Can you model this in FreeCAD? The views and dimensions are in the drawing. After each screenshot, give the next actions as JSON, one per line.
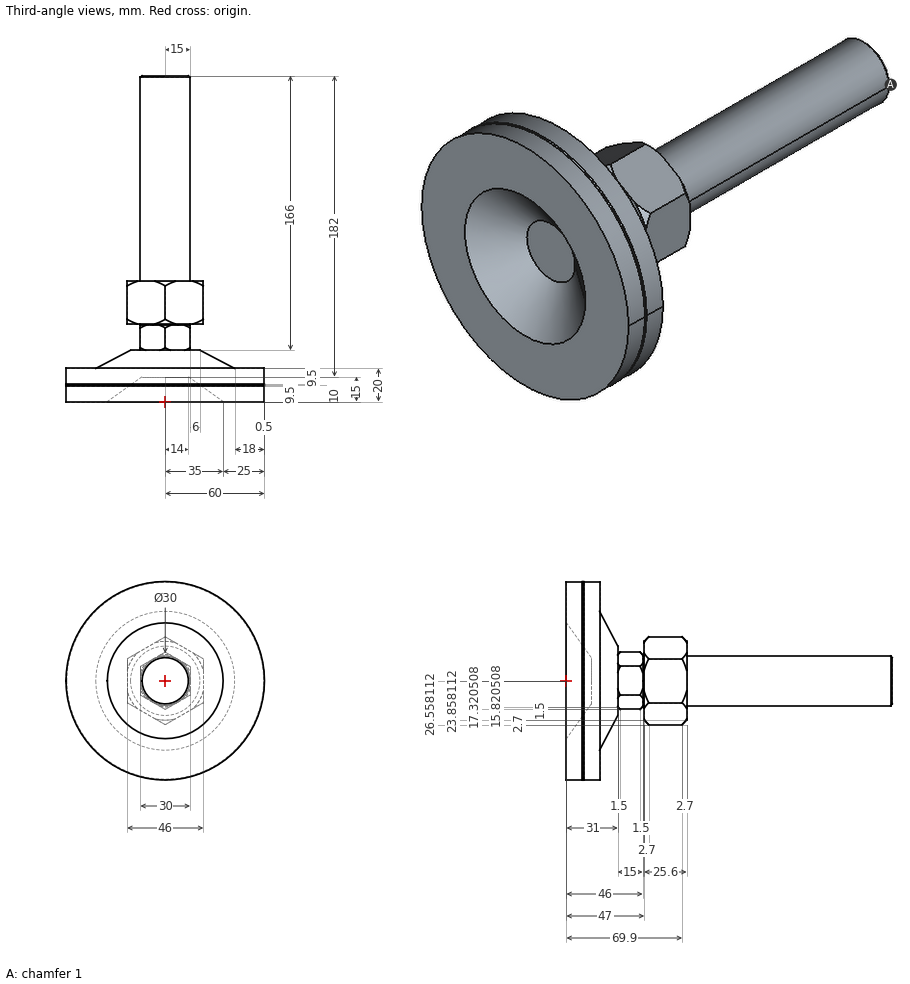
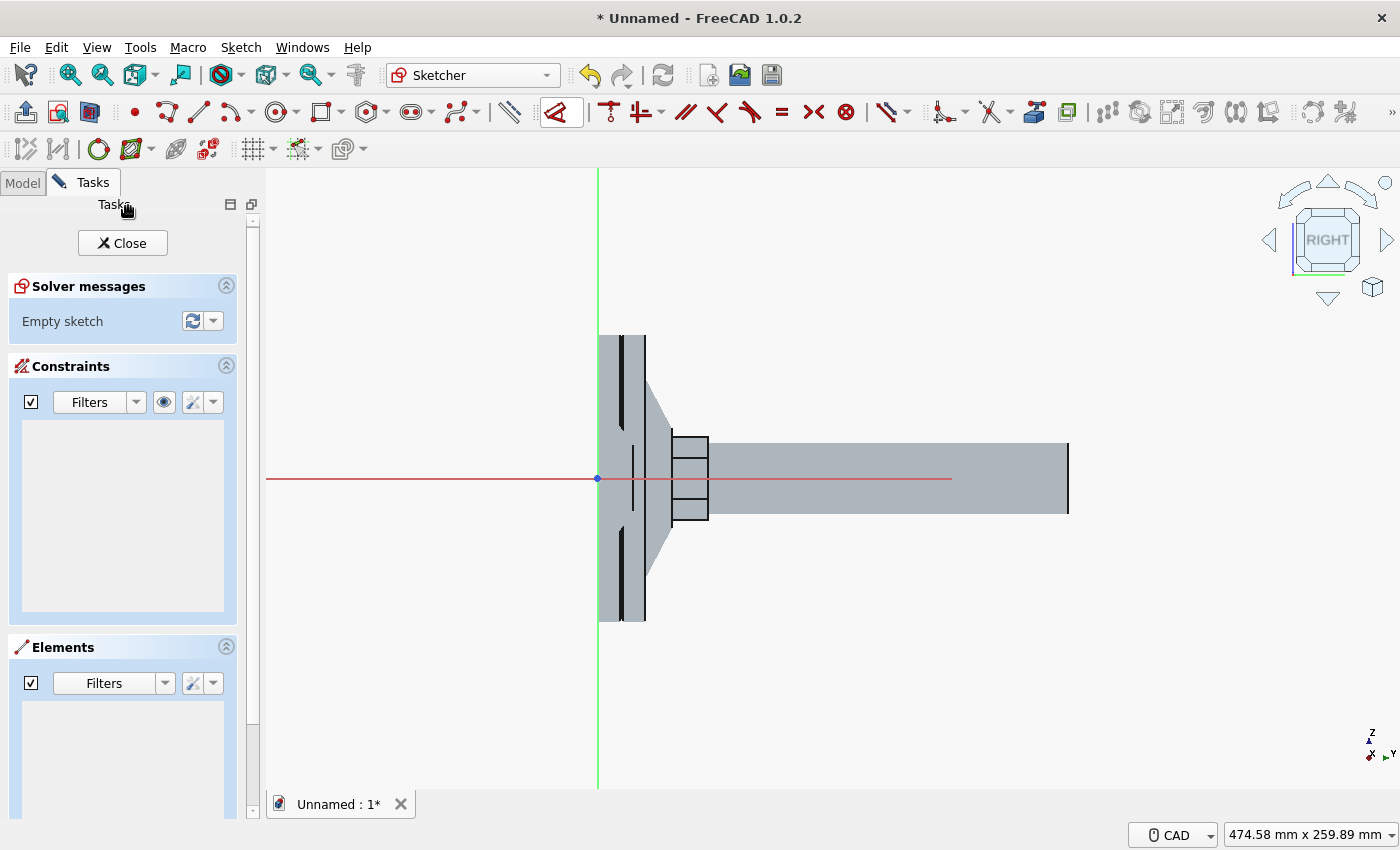
{"action": "scroll", "coordinate": [686, 520], "scroll_direction": "up", "scroll_amount": 15}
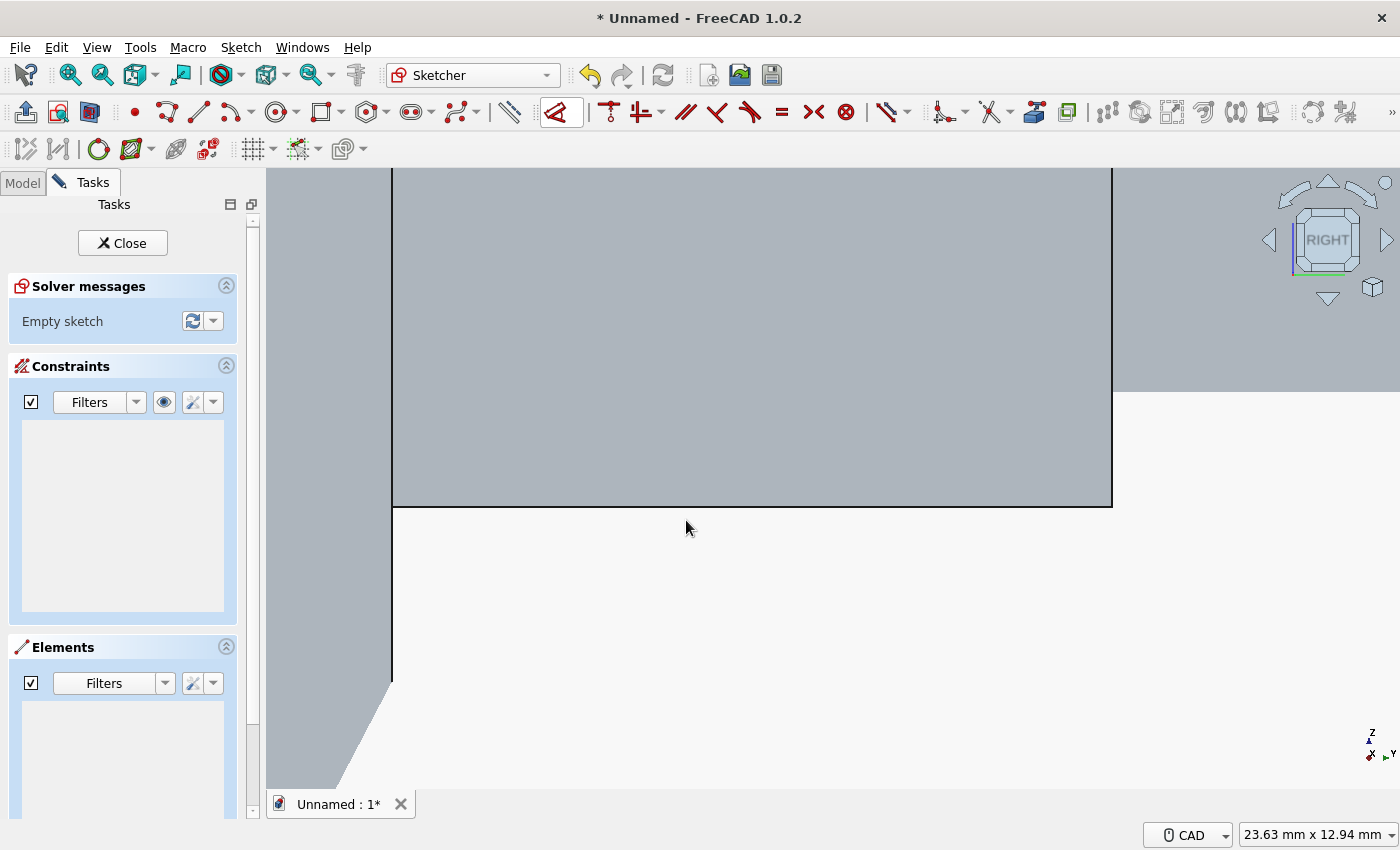
{"action": "key", "text": "g m"}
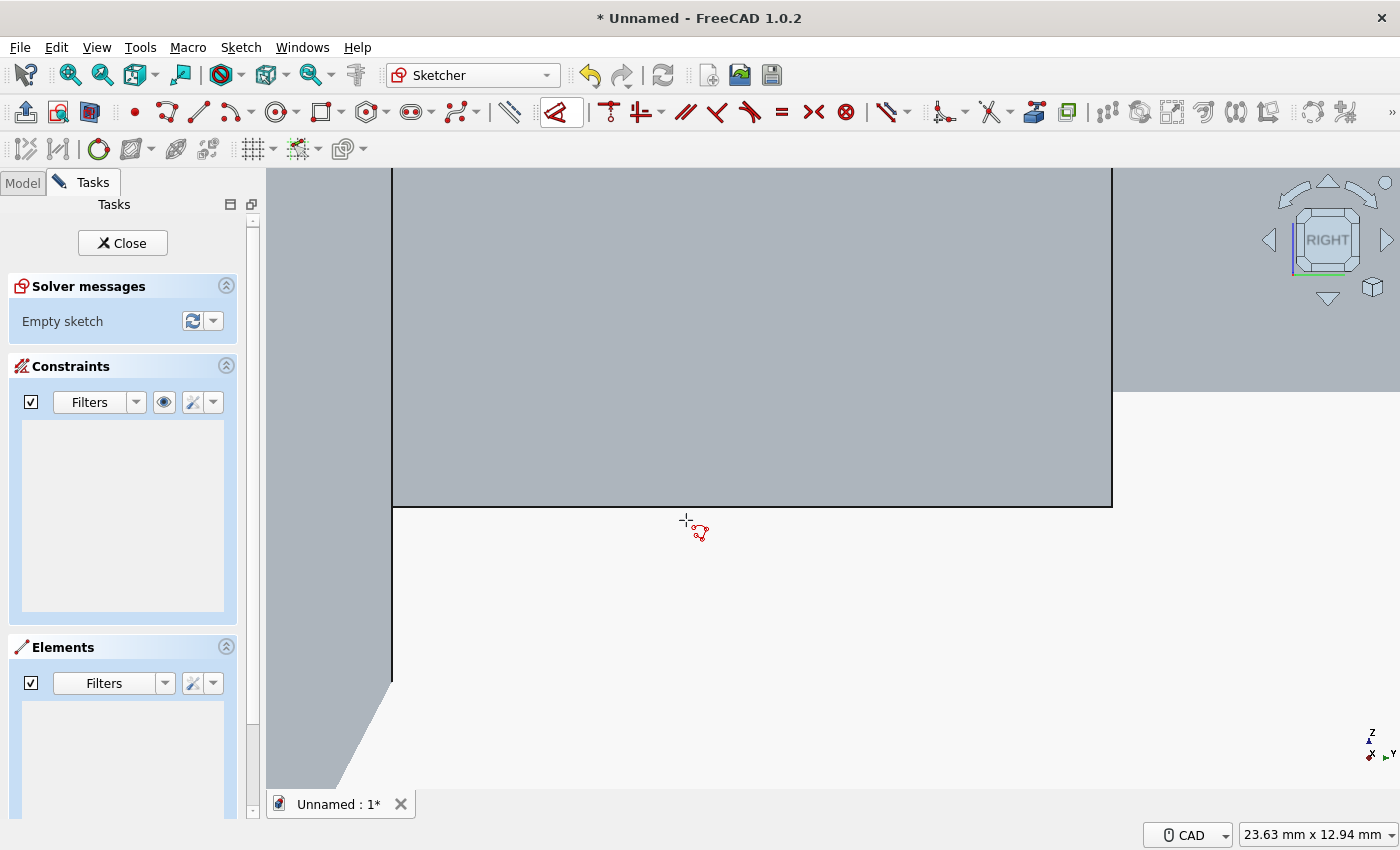
{"action": "left_click", "coordinate": [392, 435]}
{"action": "left_click", "coordinate": [392, 507]}
{"action": "left_click", "coordinate": [464, 507]}
{"action": "left_click", "coordinate": [392, 436]}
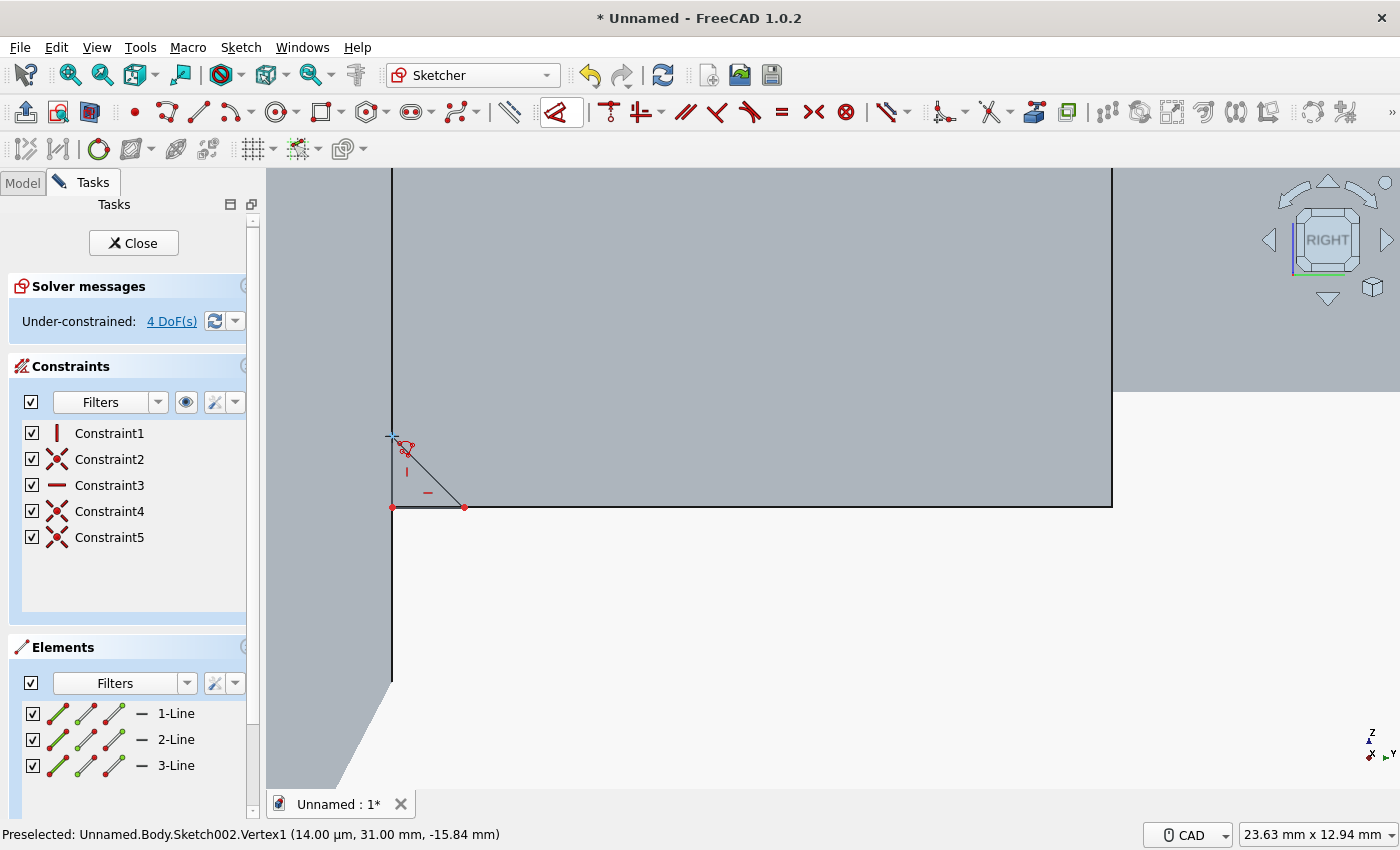
{"action": "left_click", "coordinate": [1040, 507]}
{"action": "left_click", "coordinate": [1112, 507]}
{"action": "left_click", "coordinate": [1112, 435]}
{"action": "left_click", "coordinate": [1040, 508]}
{"action": "key", "text": "Escape"}
{"action": "key", "text": "Escape"}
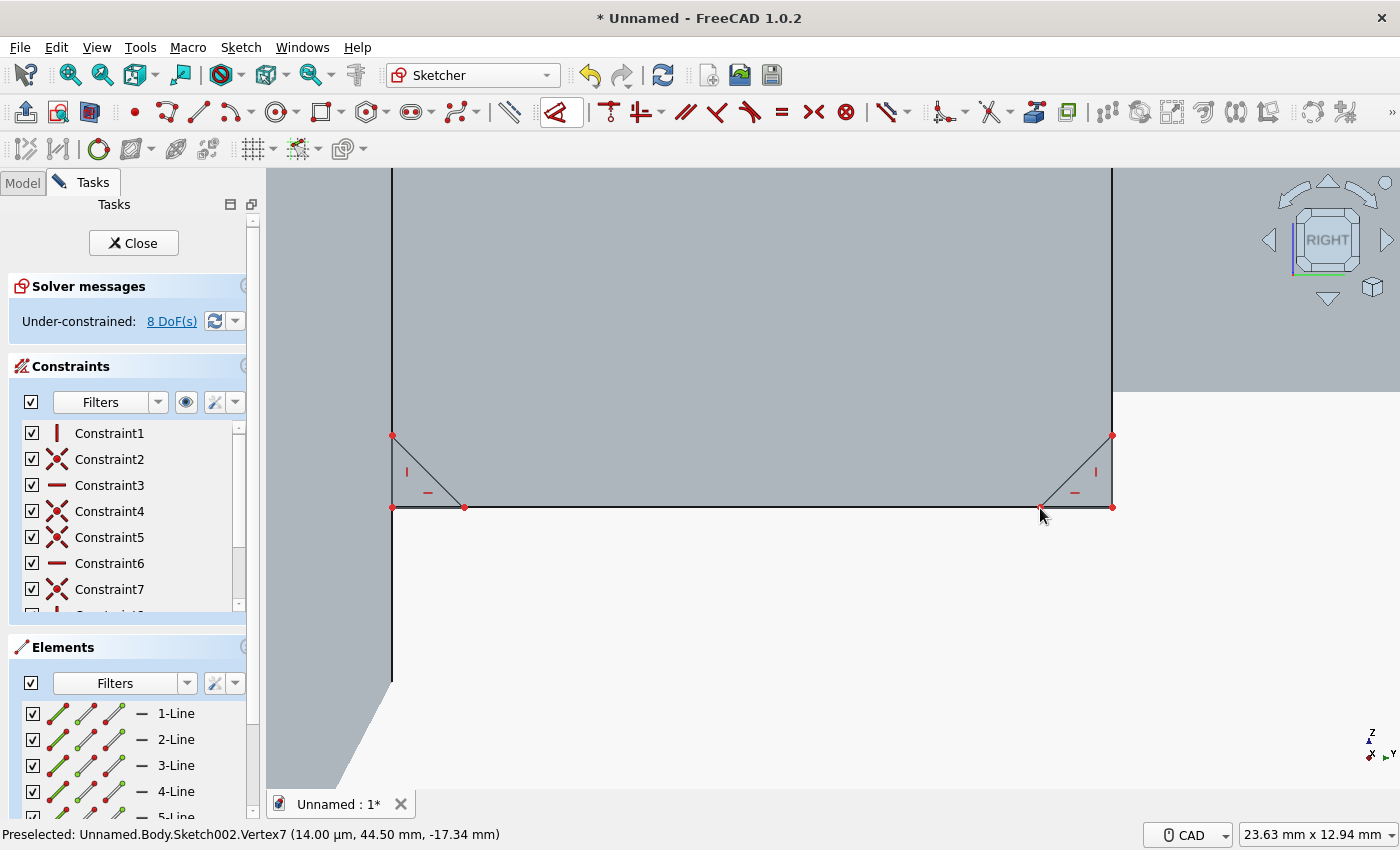
{"action": "left_click", "coordinate": [392, 458]}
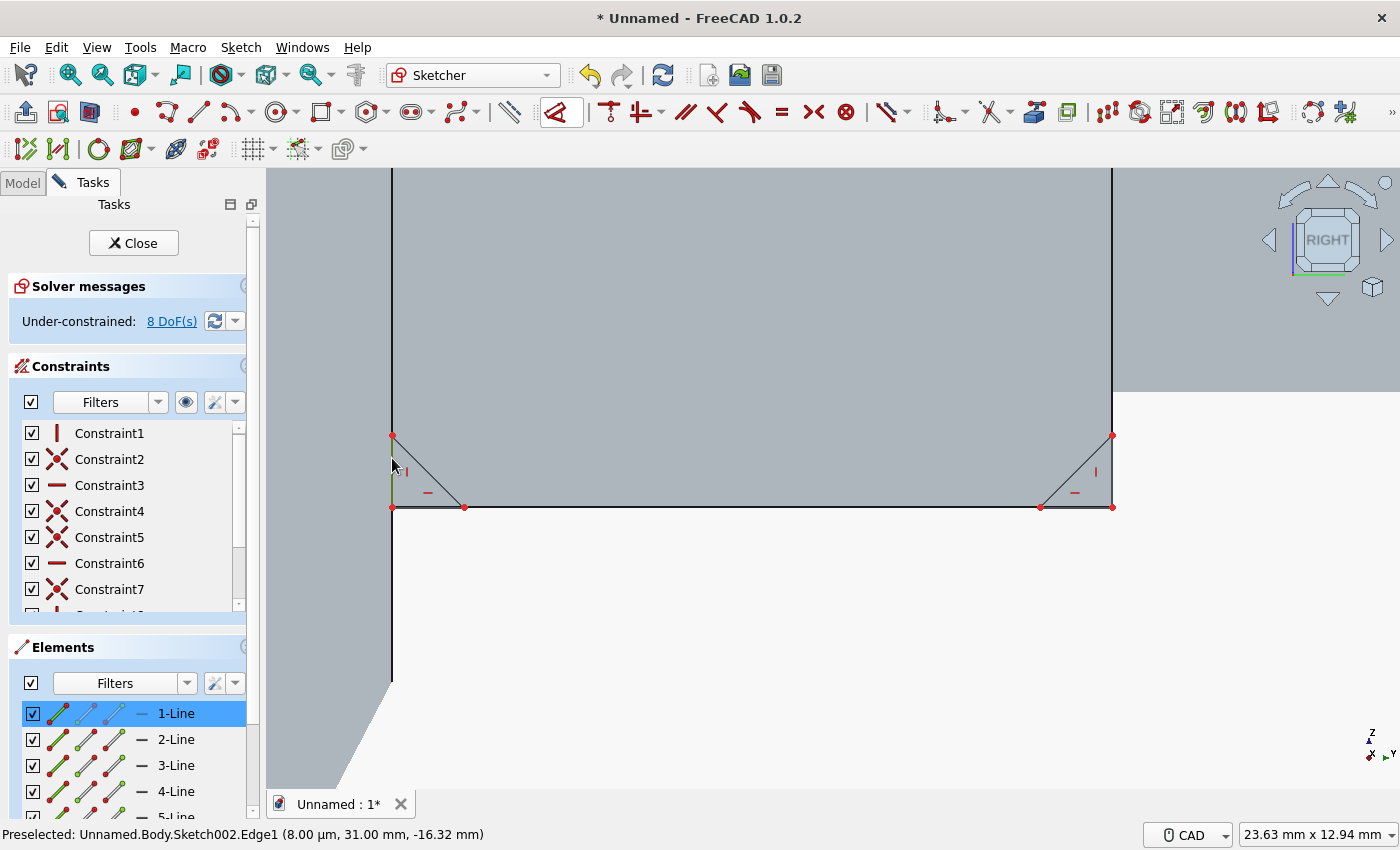
{"action": "key", "text": "i"}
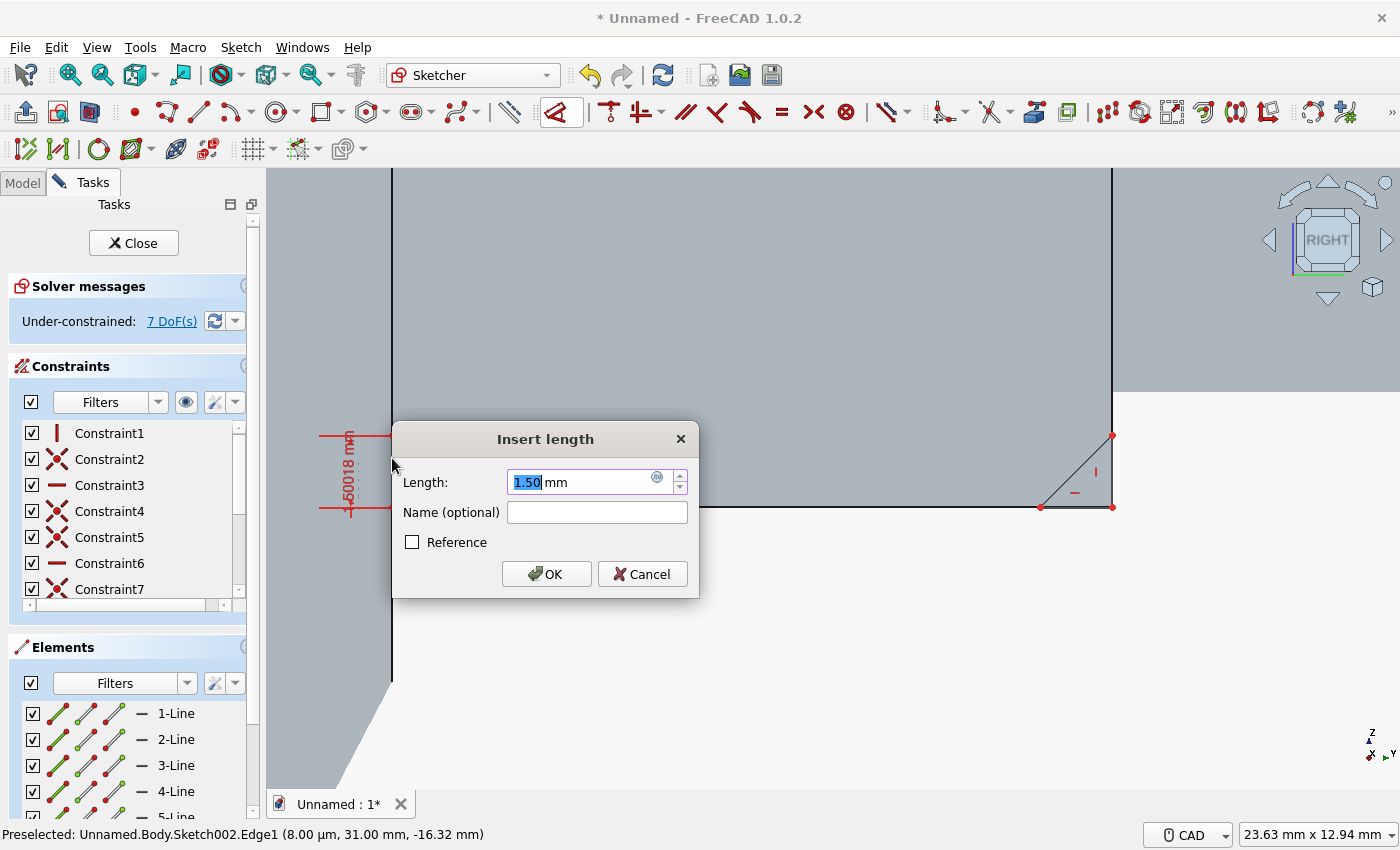
{"action": "type", "text": "1.5"}
{"action": "key", "text": "Return"}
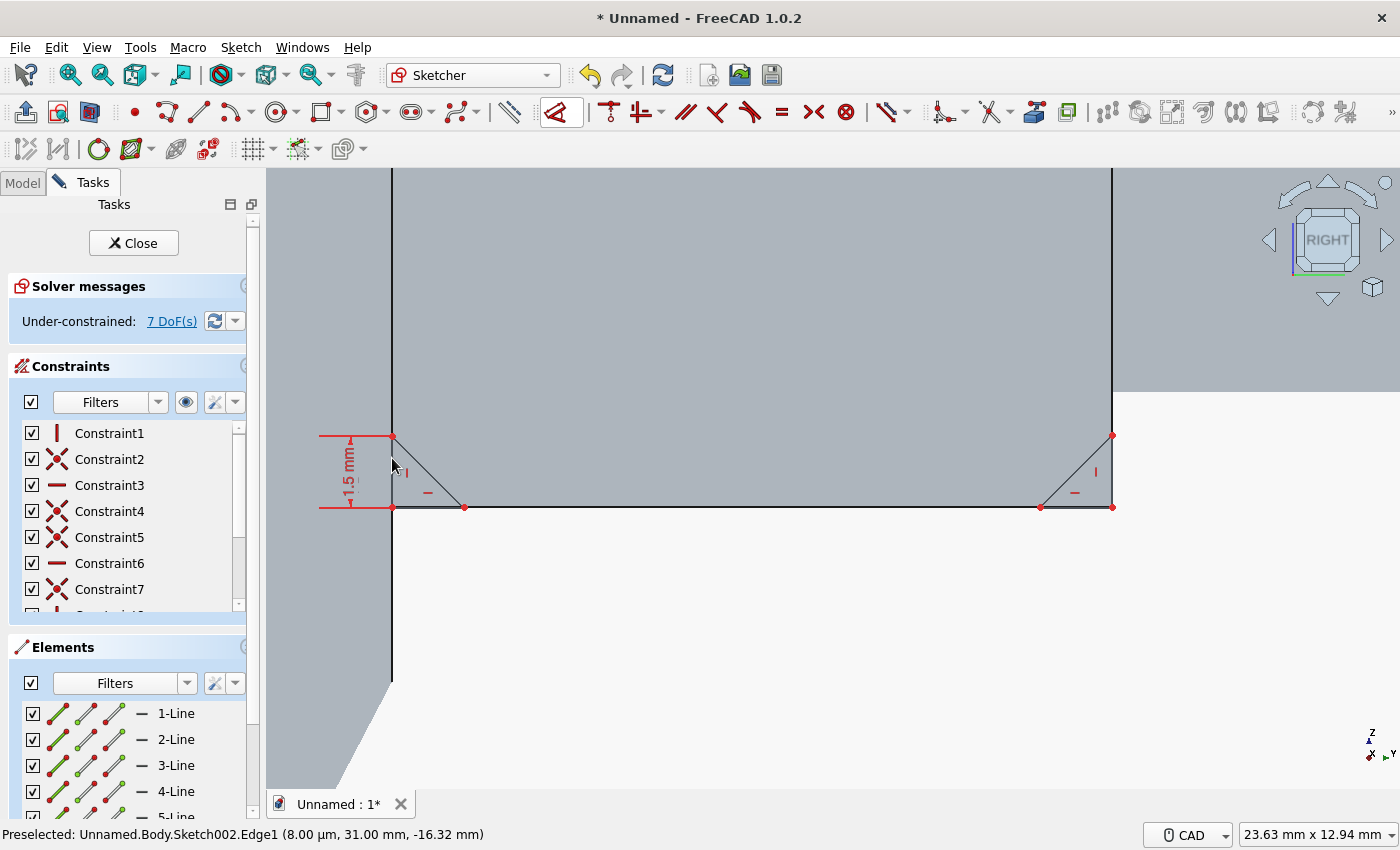
{"action": "left_click", "coordinate": [414, 508]}